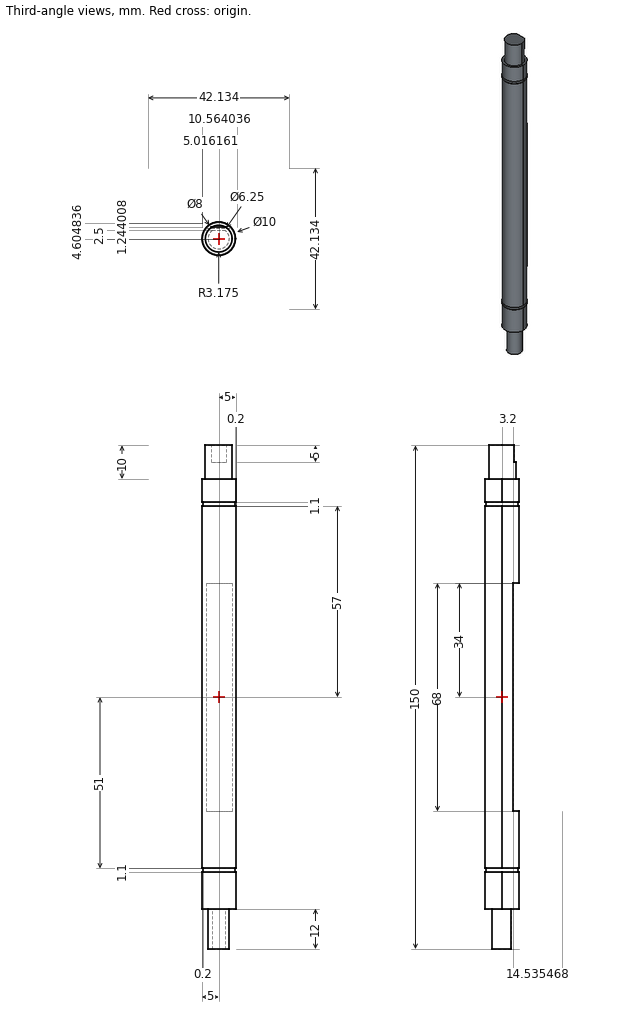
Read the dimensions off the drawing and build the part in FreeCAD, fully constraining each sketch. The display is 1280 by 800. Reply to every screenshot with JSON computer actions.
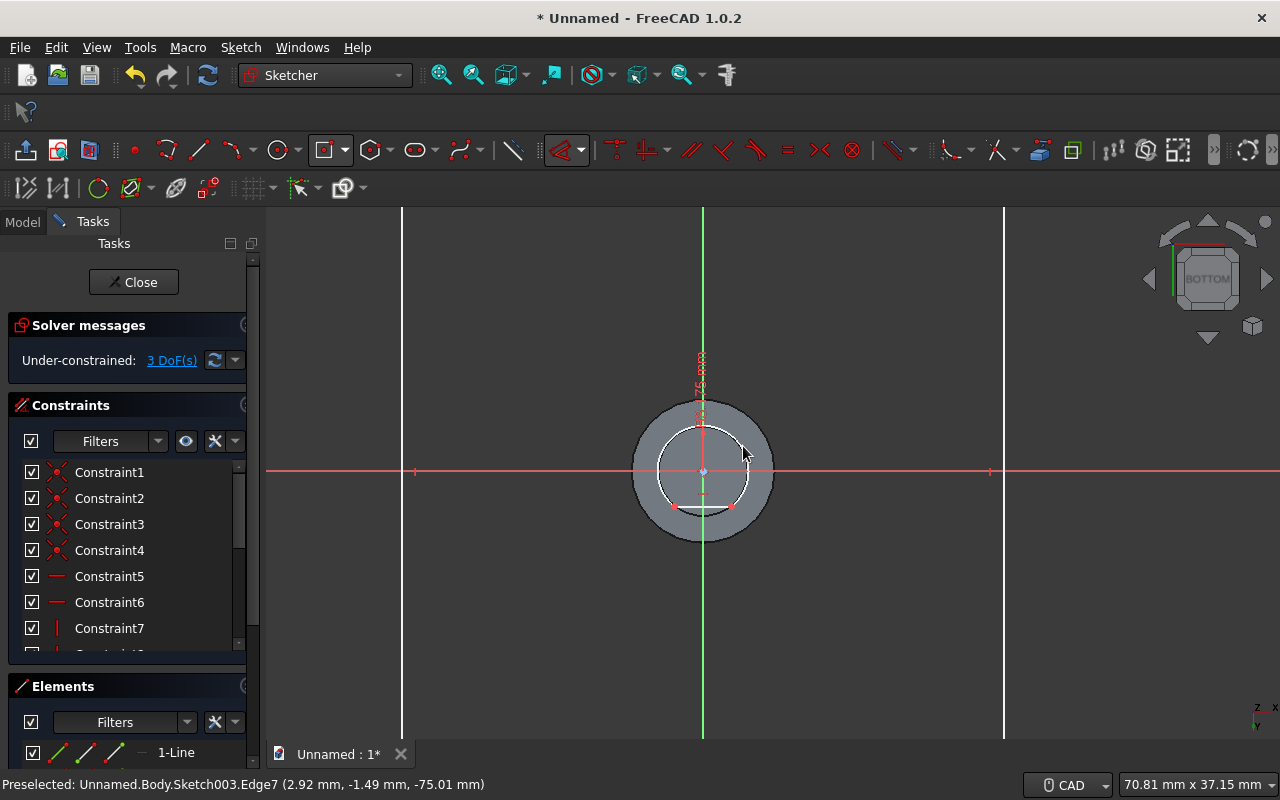
{"action": "left_click", "coordinate": [675, 507]}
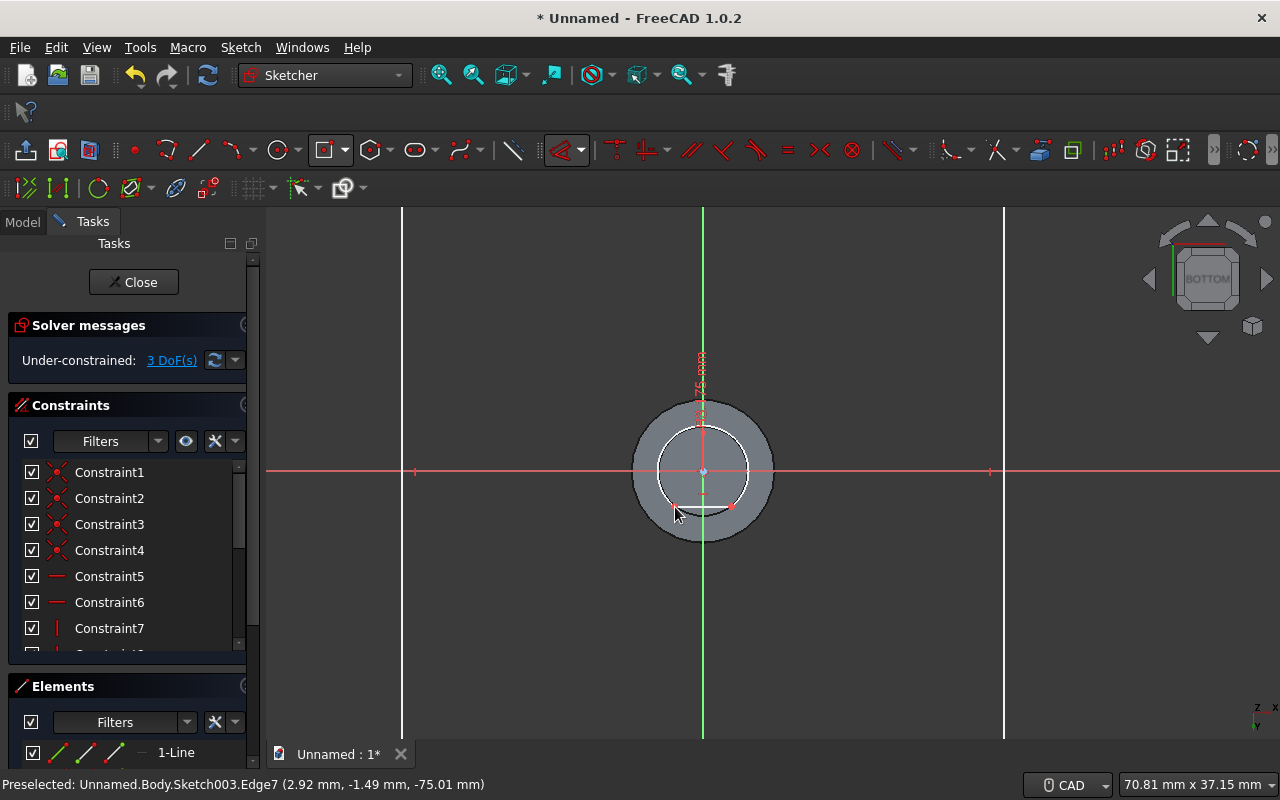
{"action": "left_click", "coordinate": [584, 150]}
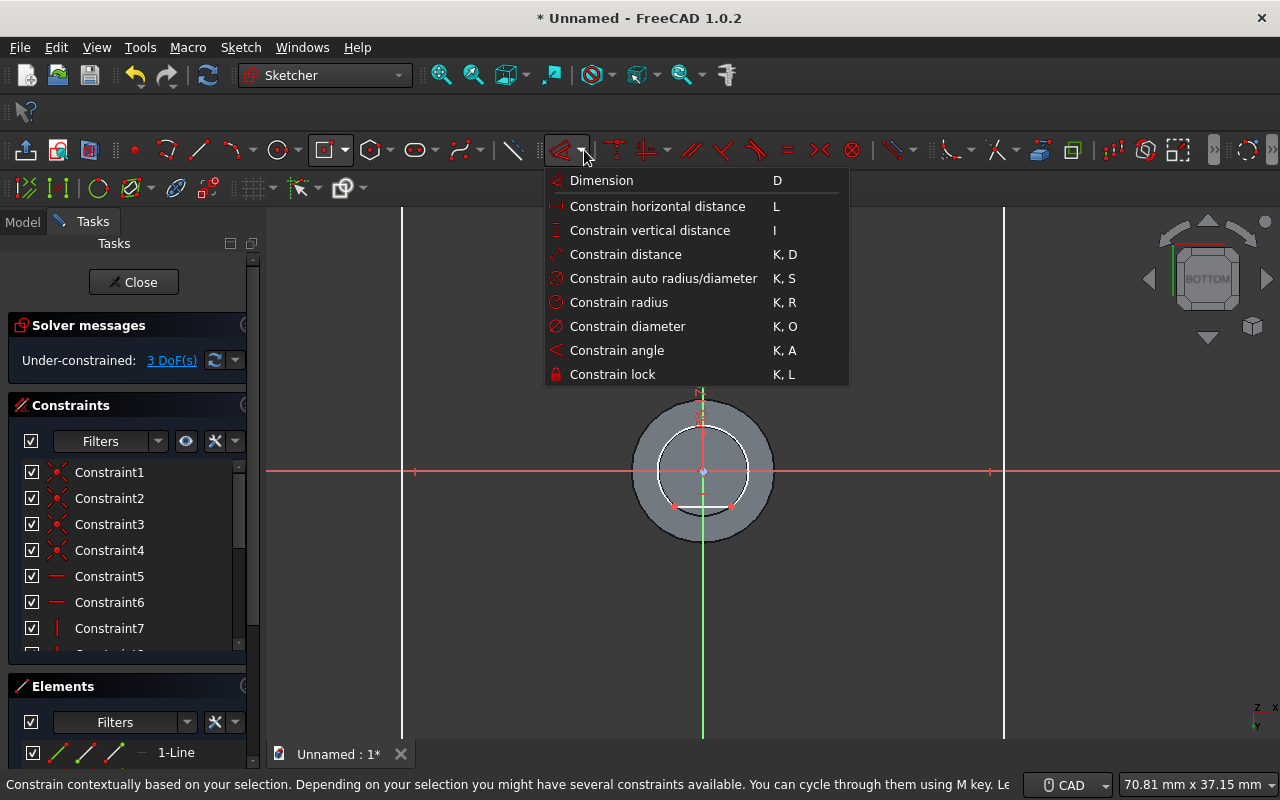
{"action": "left_click", "coordinate": [697, 230]}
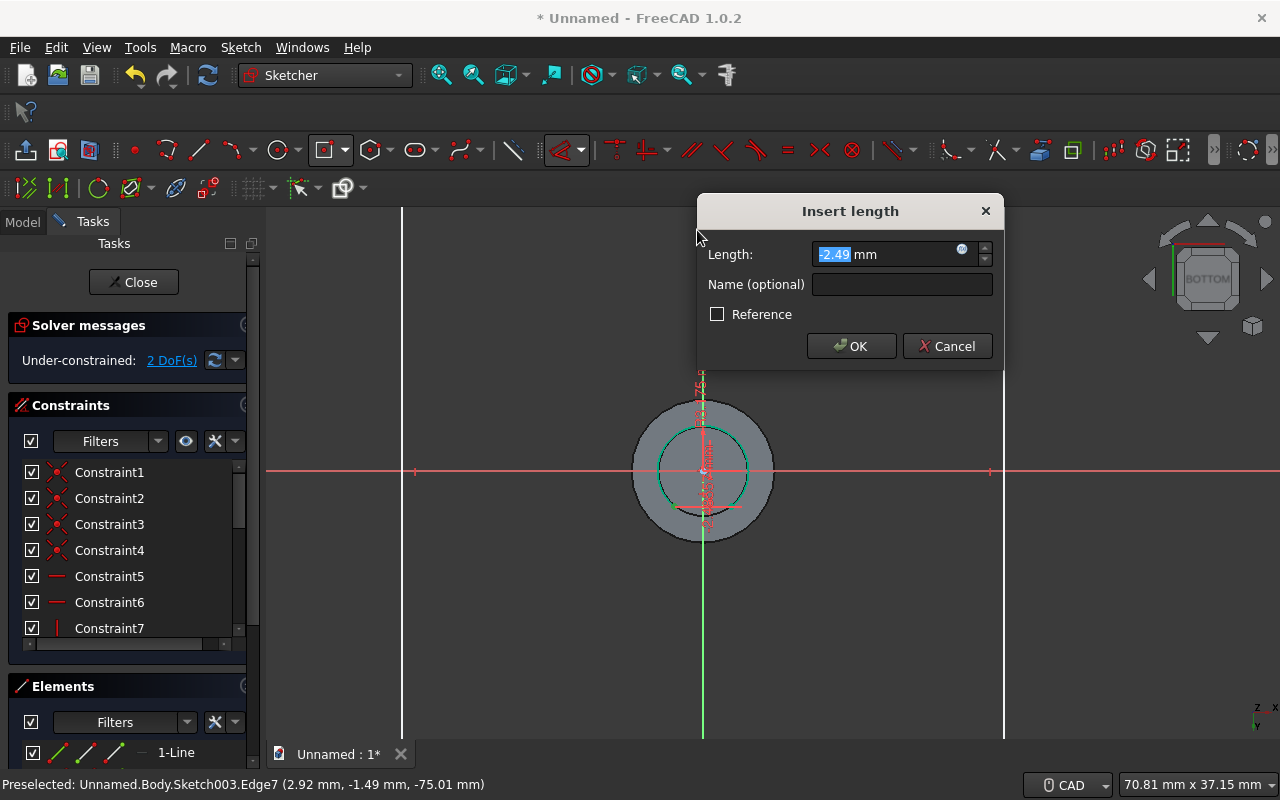
{"action": "type", "text": "-2.5"}
{"action": "key", "text": "Return"}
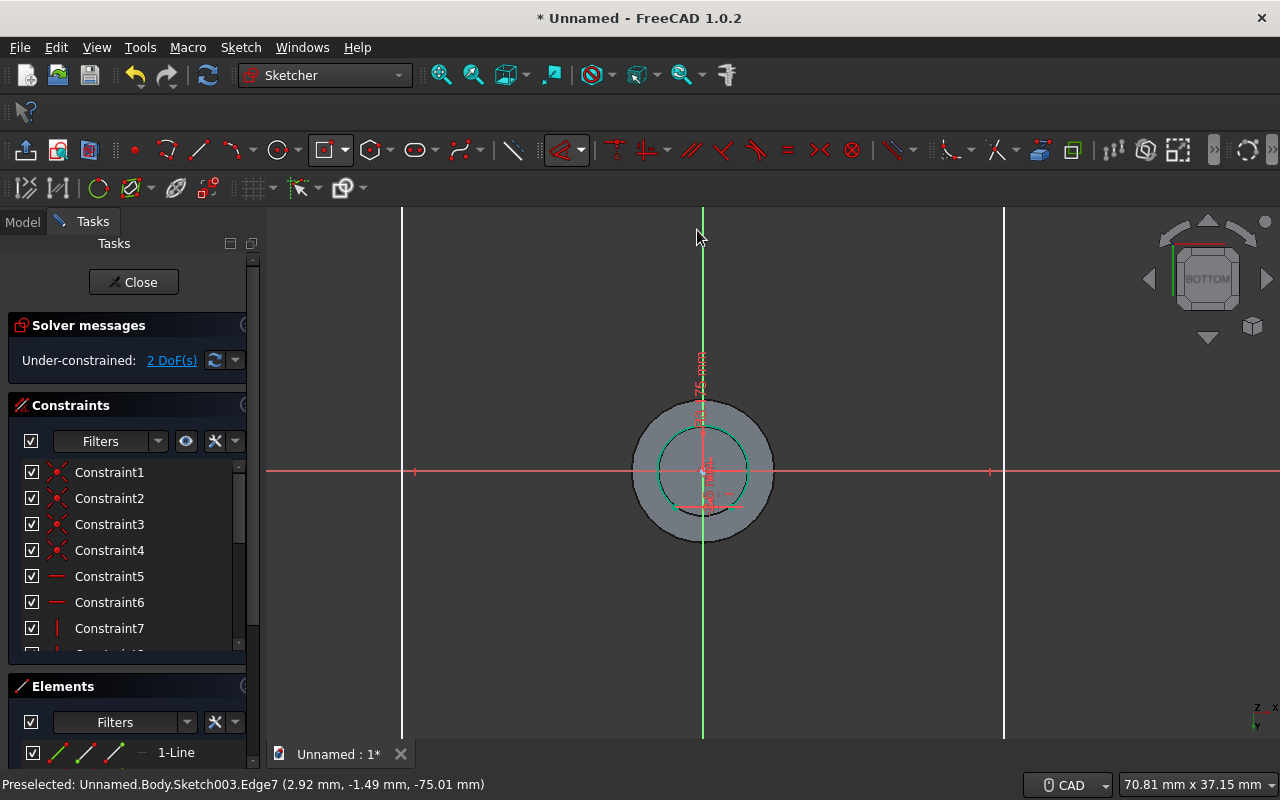
{"action": "scroll", "coordinate": [706, 475], "scroll_direction": "down", "scroll_amount": 3}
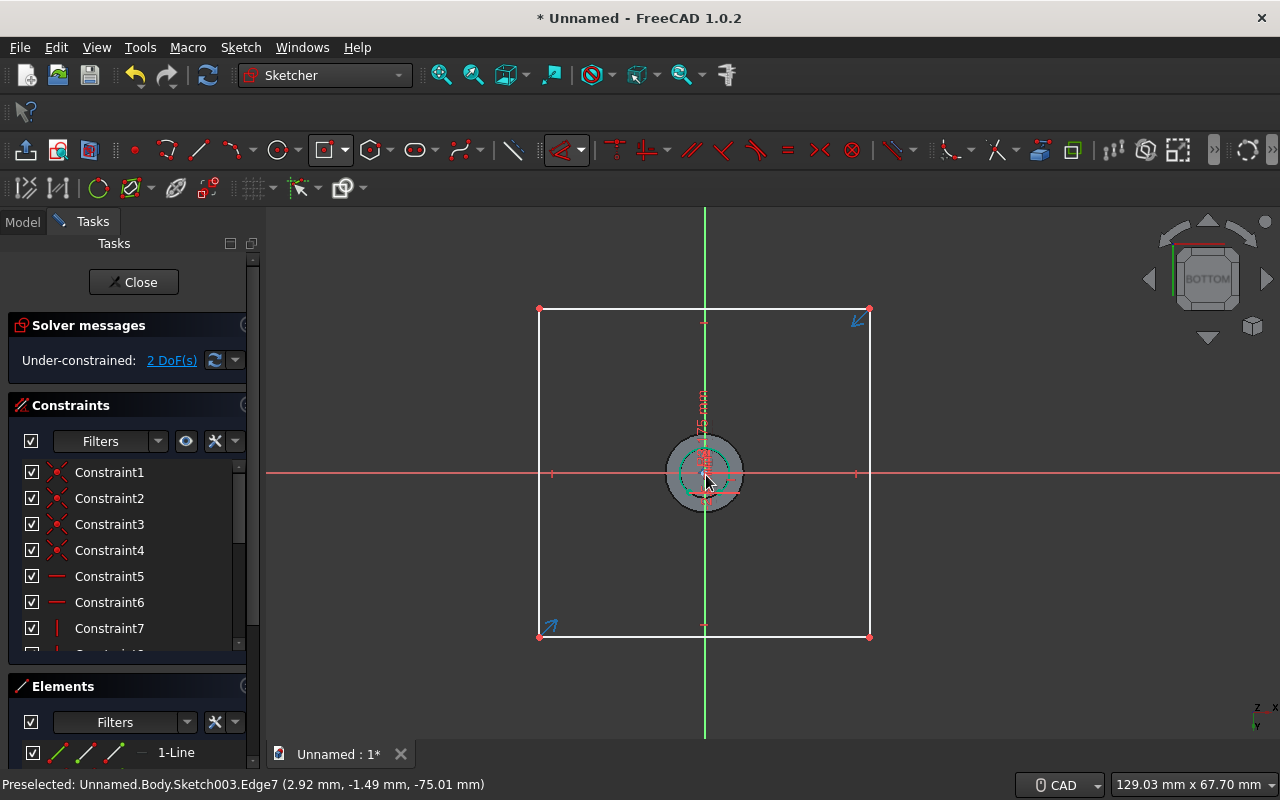
{"action": "left_click", "coordinate": [638, 637]}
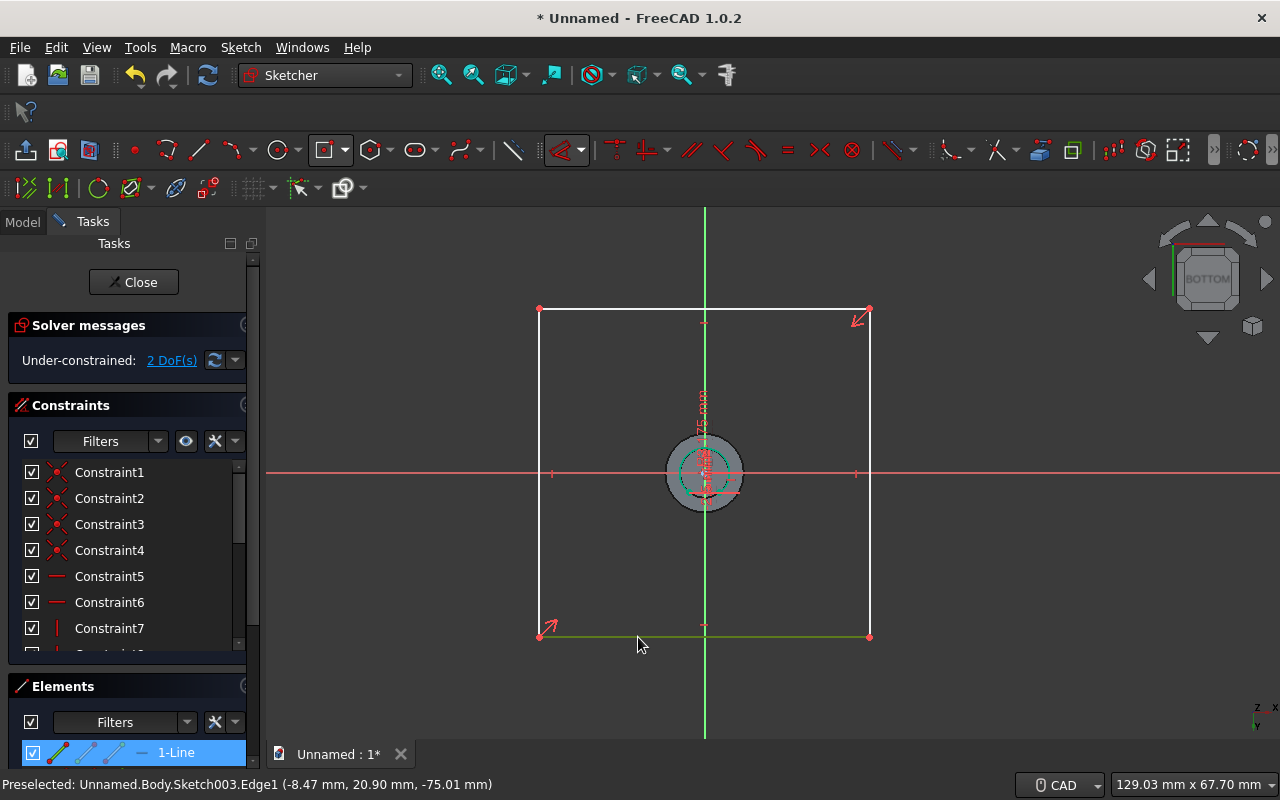
{"action": "key", "text": "l"}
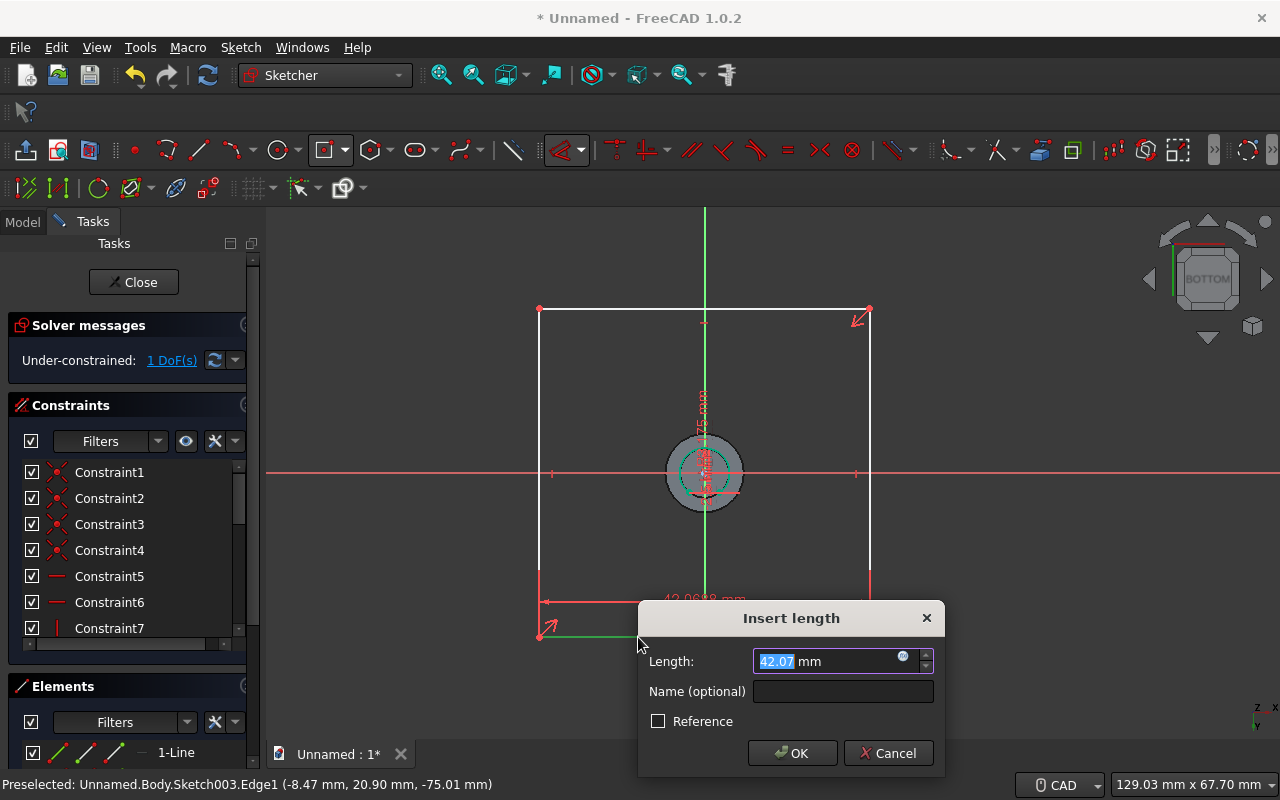
{"action": "type", "text": "42.134"}
{"action": "key", "text": "Return"}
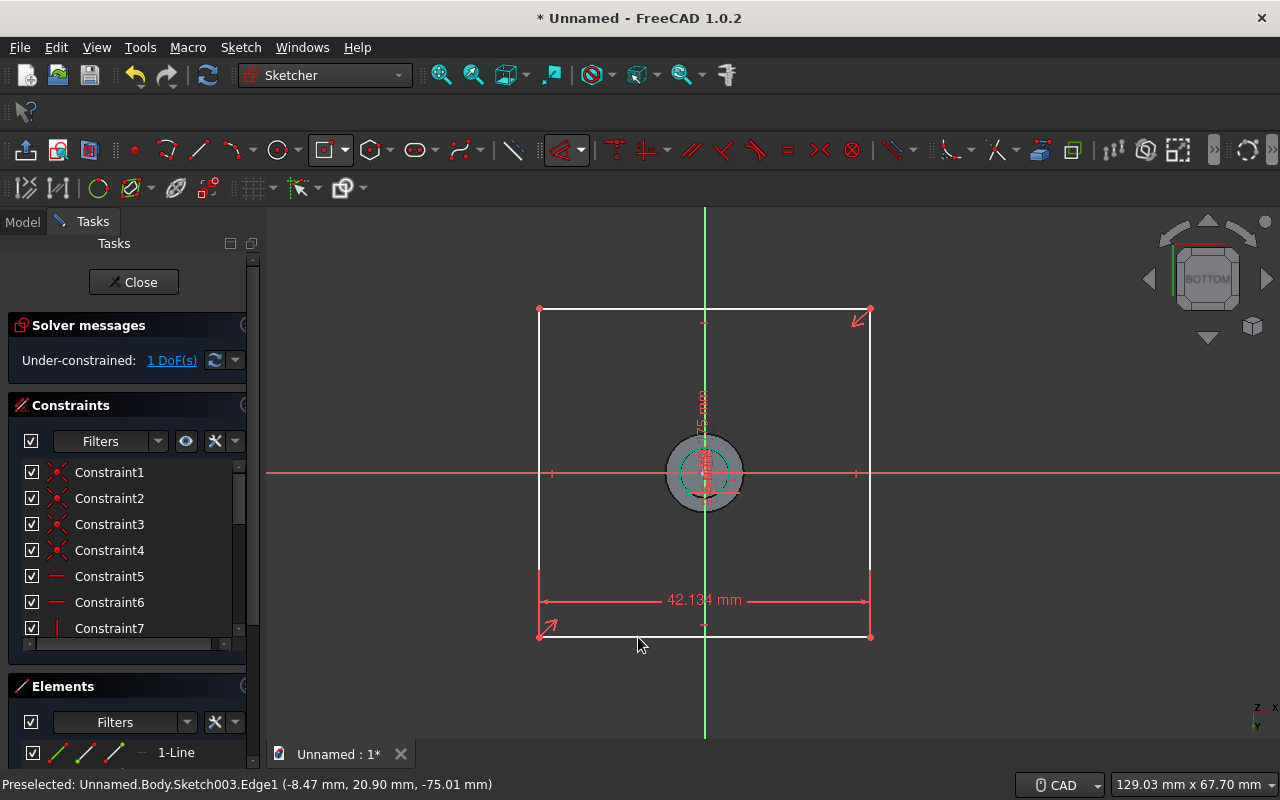
{"action": "left_click", "coordinate": [870, 539]}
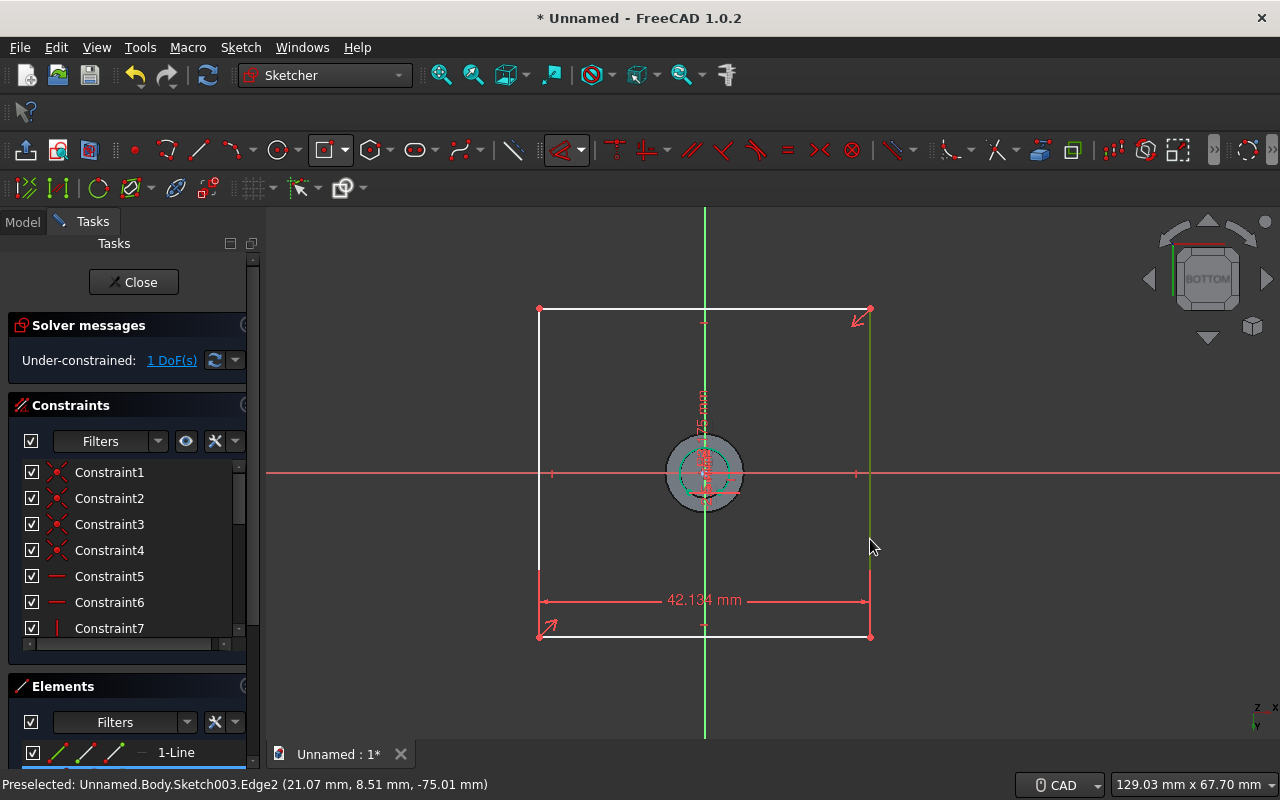
{"action": "left_click", "coordinate": [584, 150]}